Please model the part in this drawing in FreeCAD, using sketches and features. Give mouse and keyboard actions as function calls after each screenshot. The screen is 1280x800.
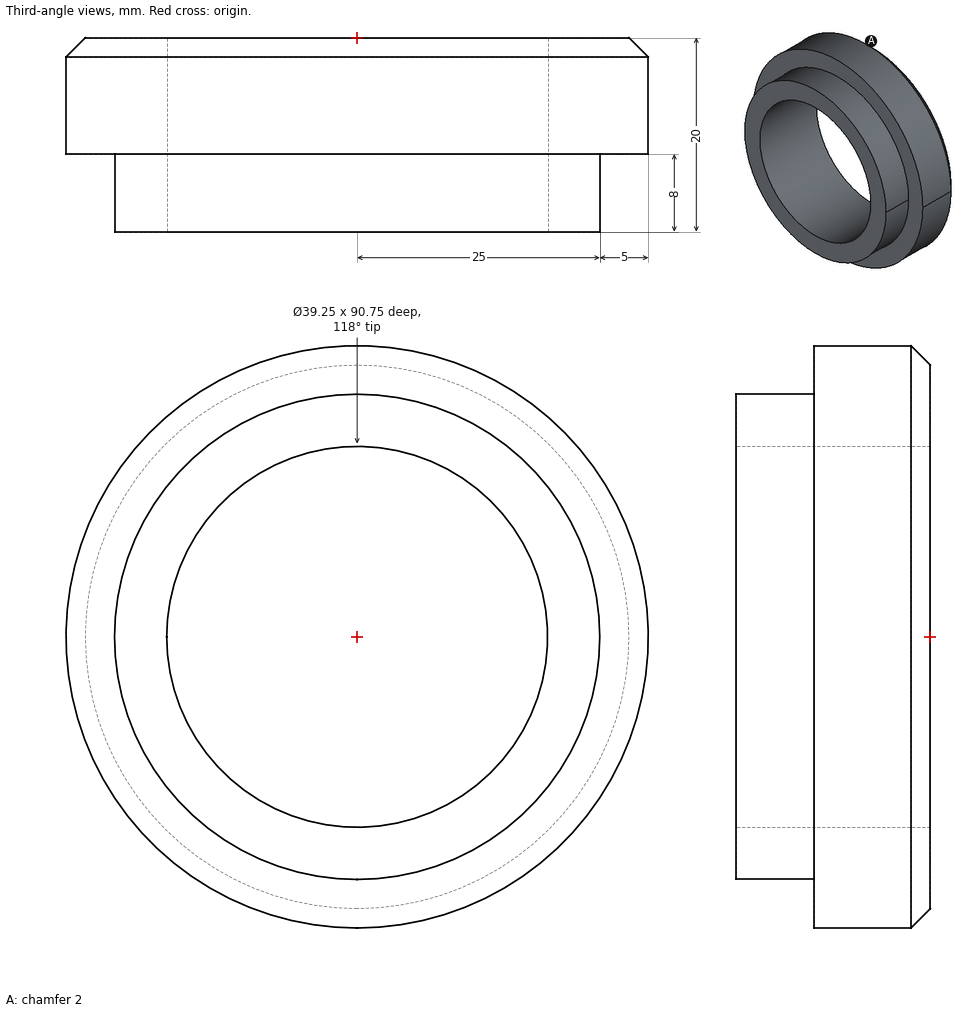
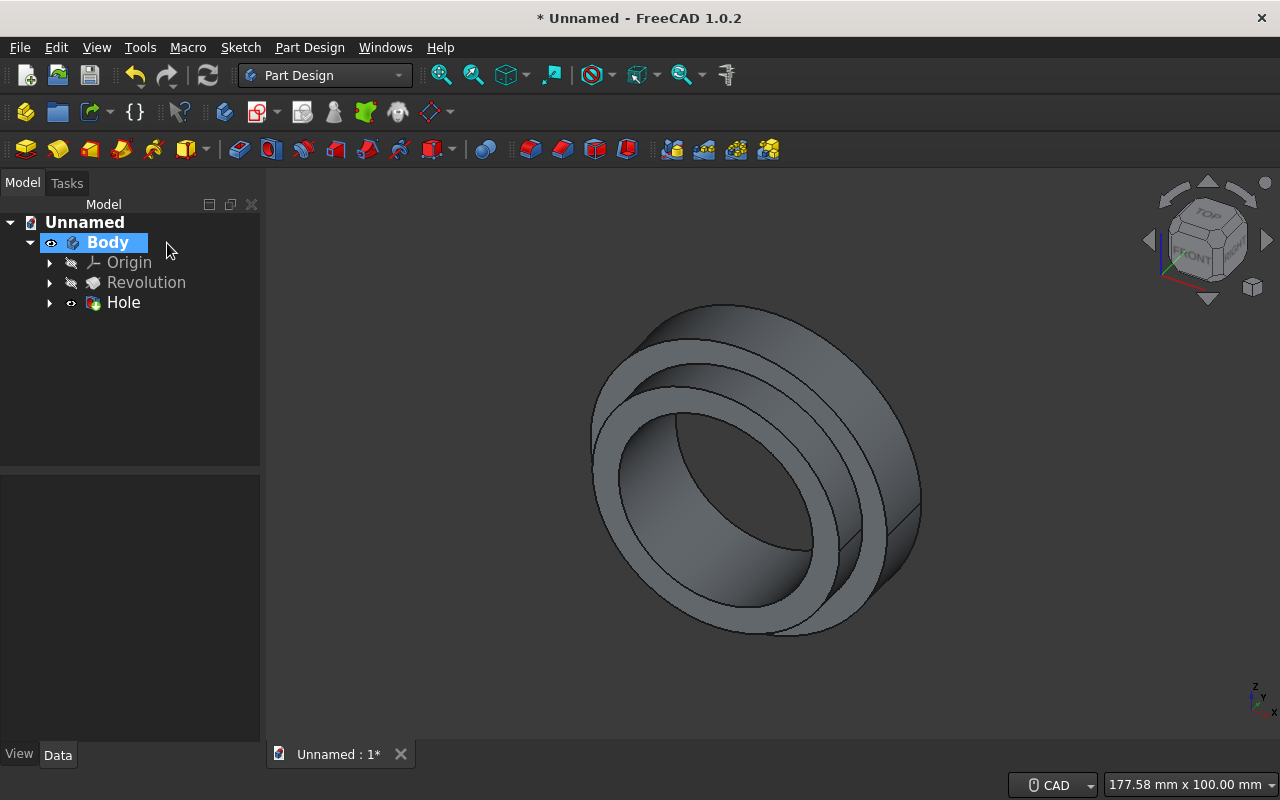
key(0)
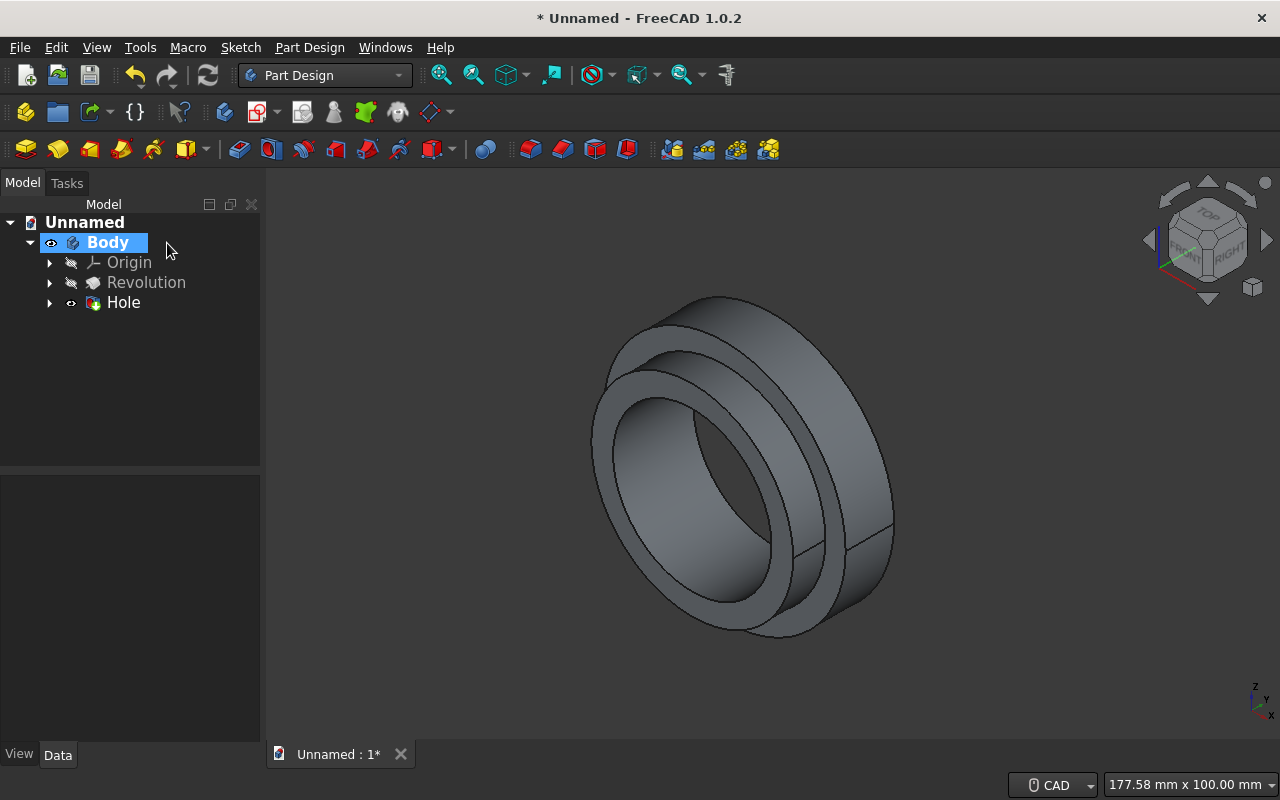
key(2)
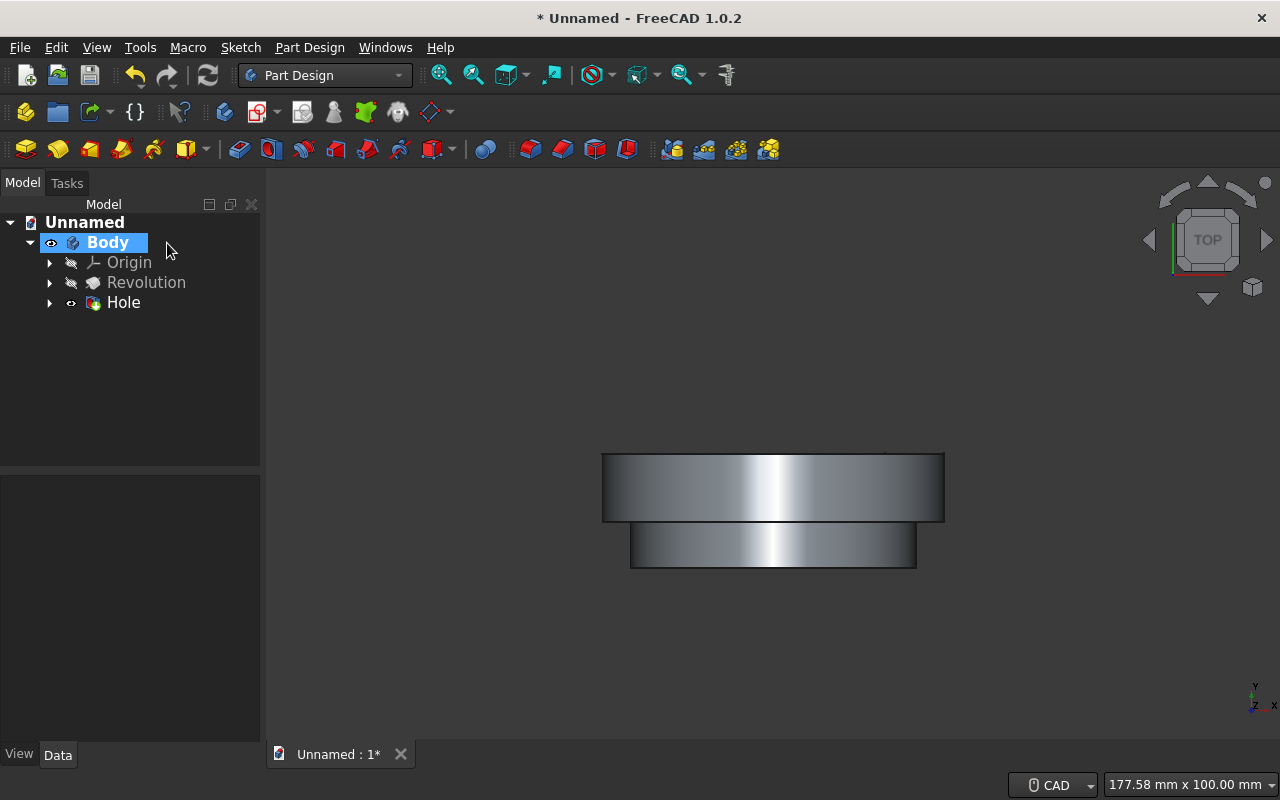
click(442, 76)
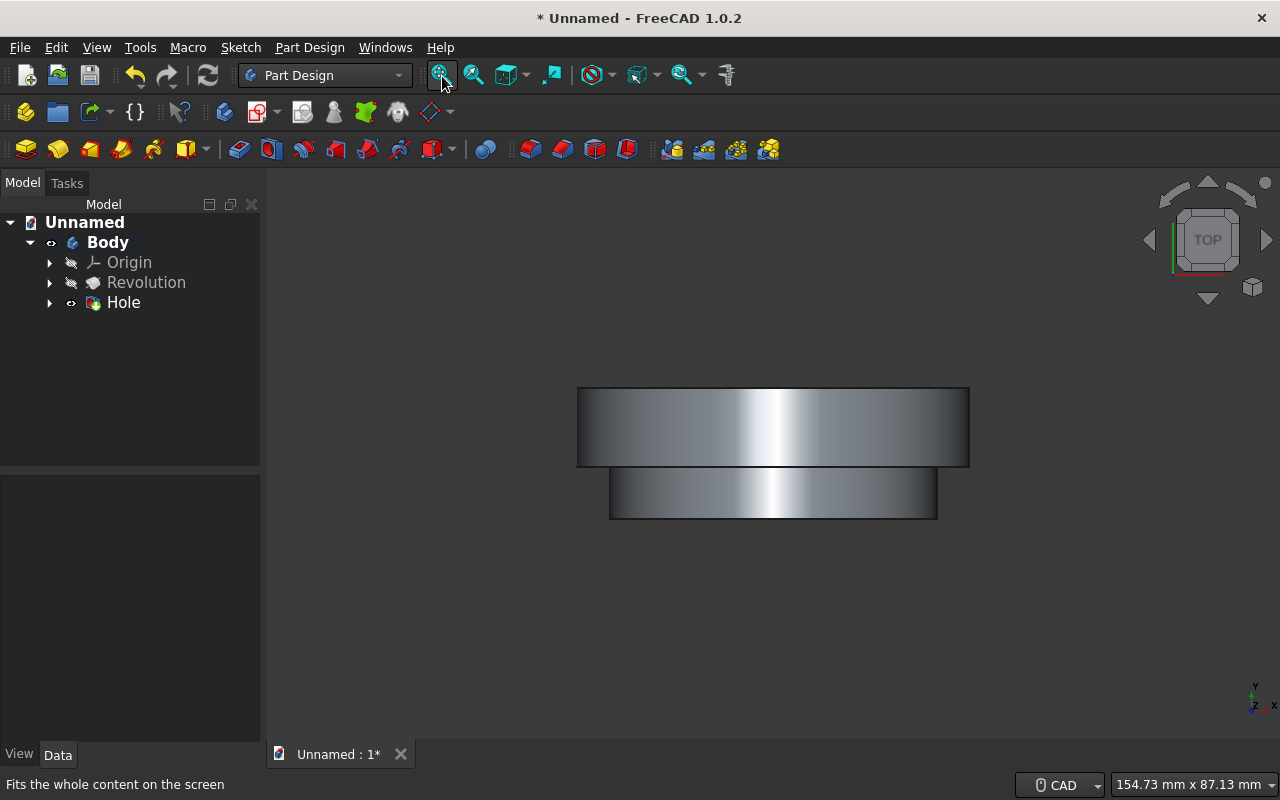
click(614, 387)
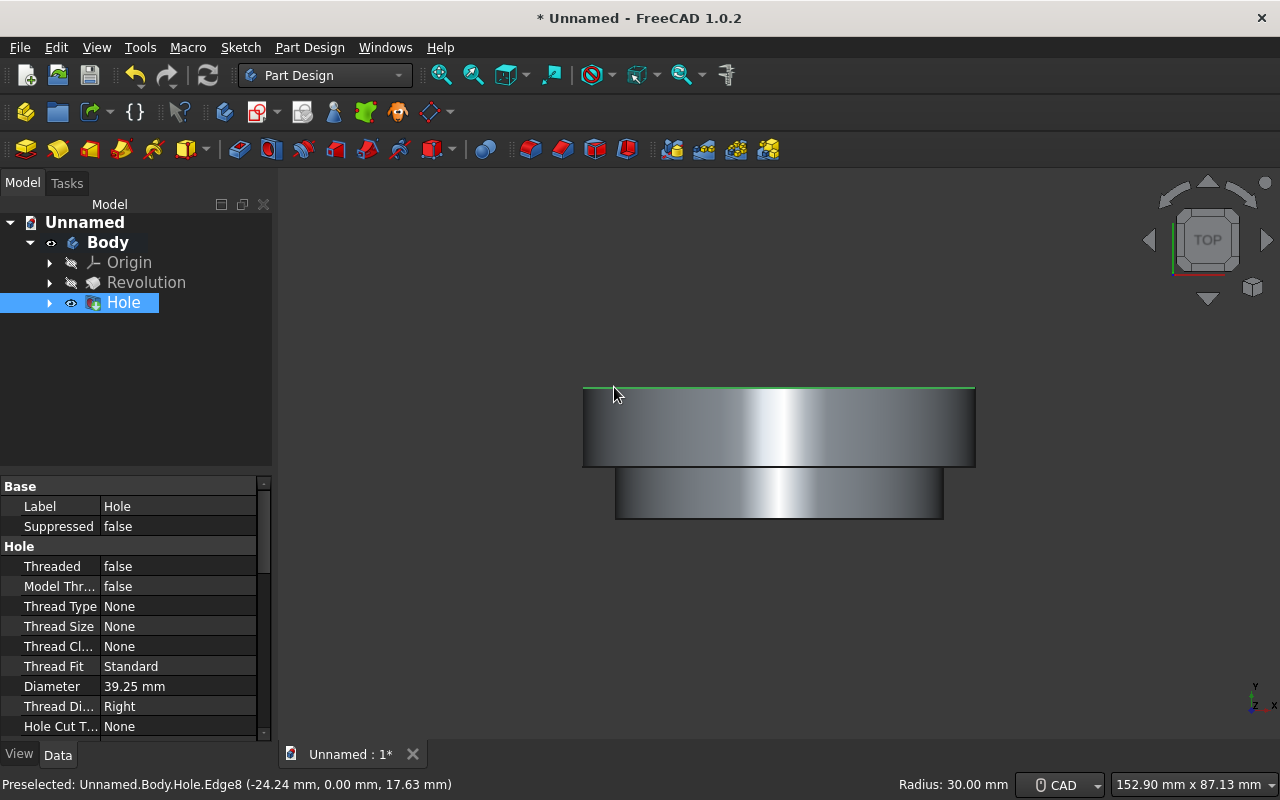
click(564, 150)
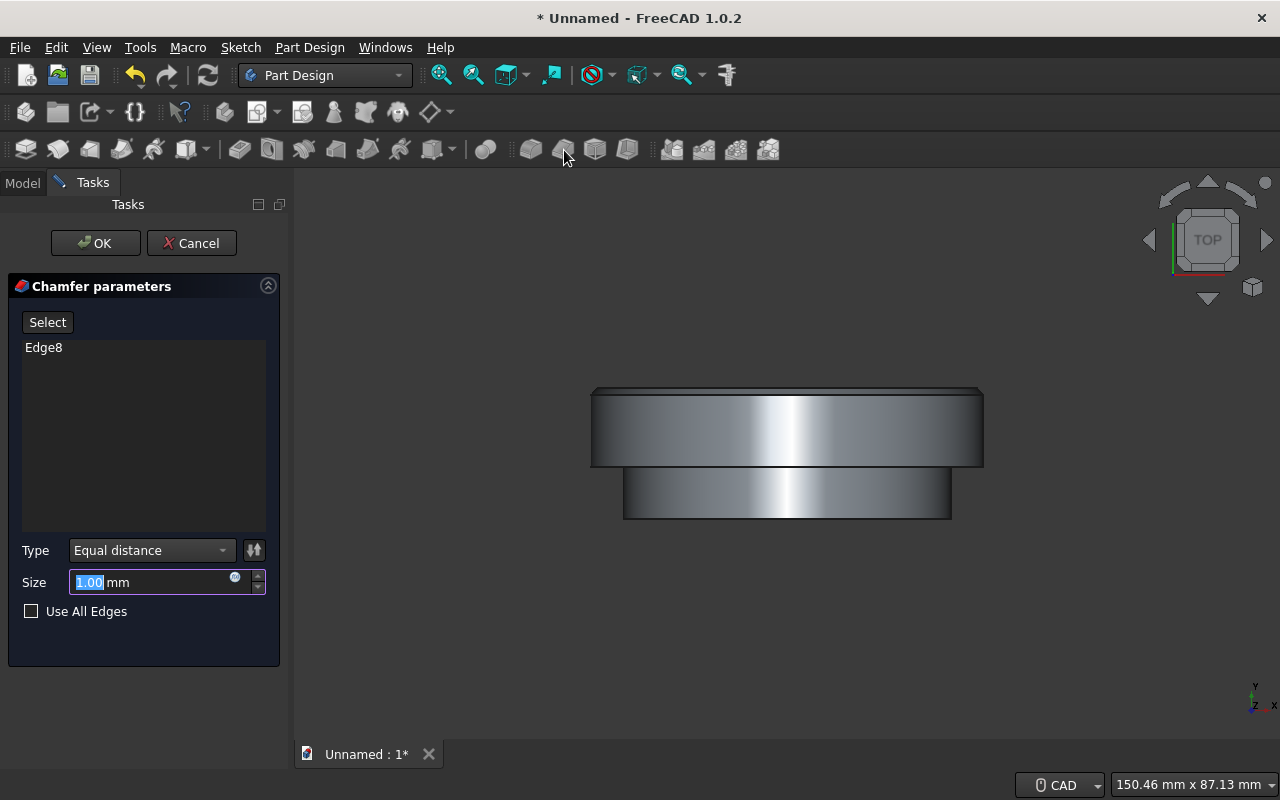
text(2)
key(Tab)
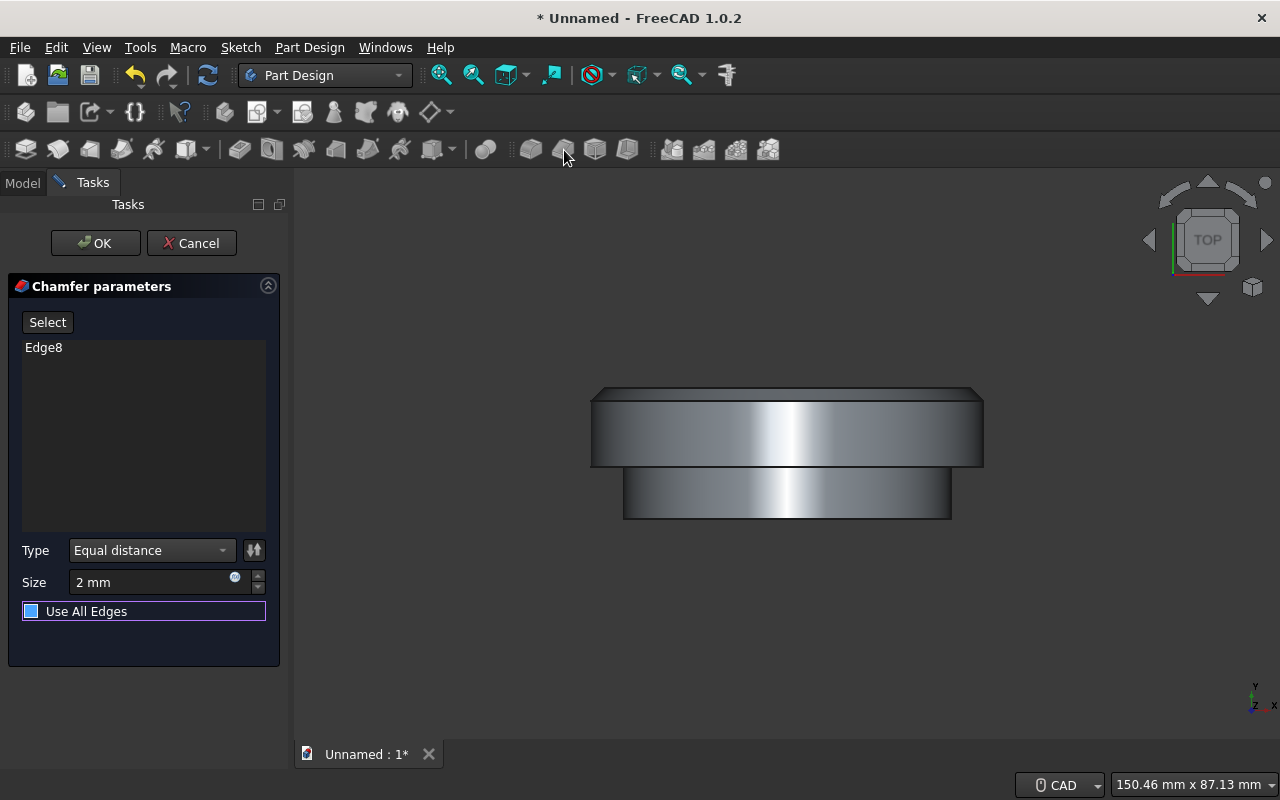
click(96, 243)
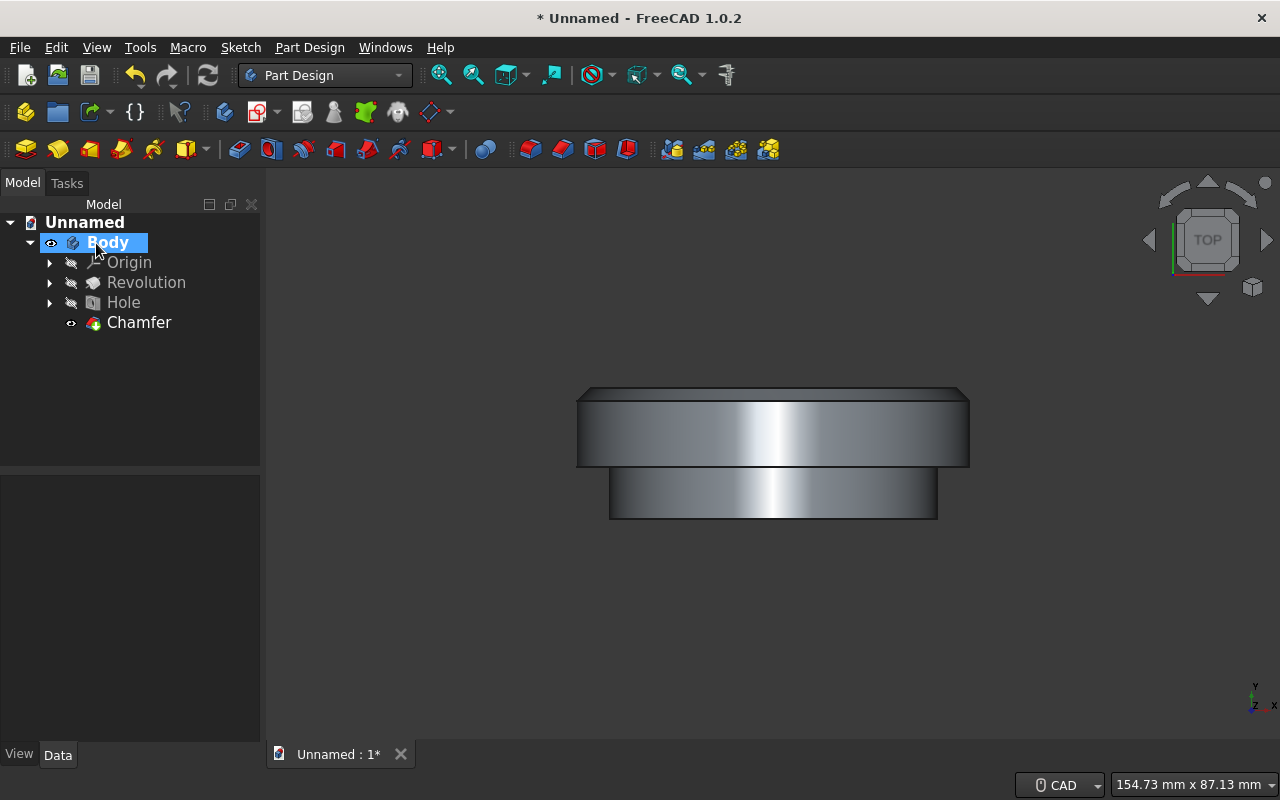
key(0)